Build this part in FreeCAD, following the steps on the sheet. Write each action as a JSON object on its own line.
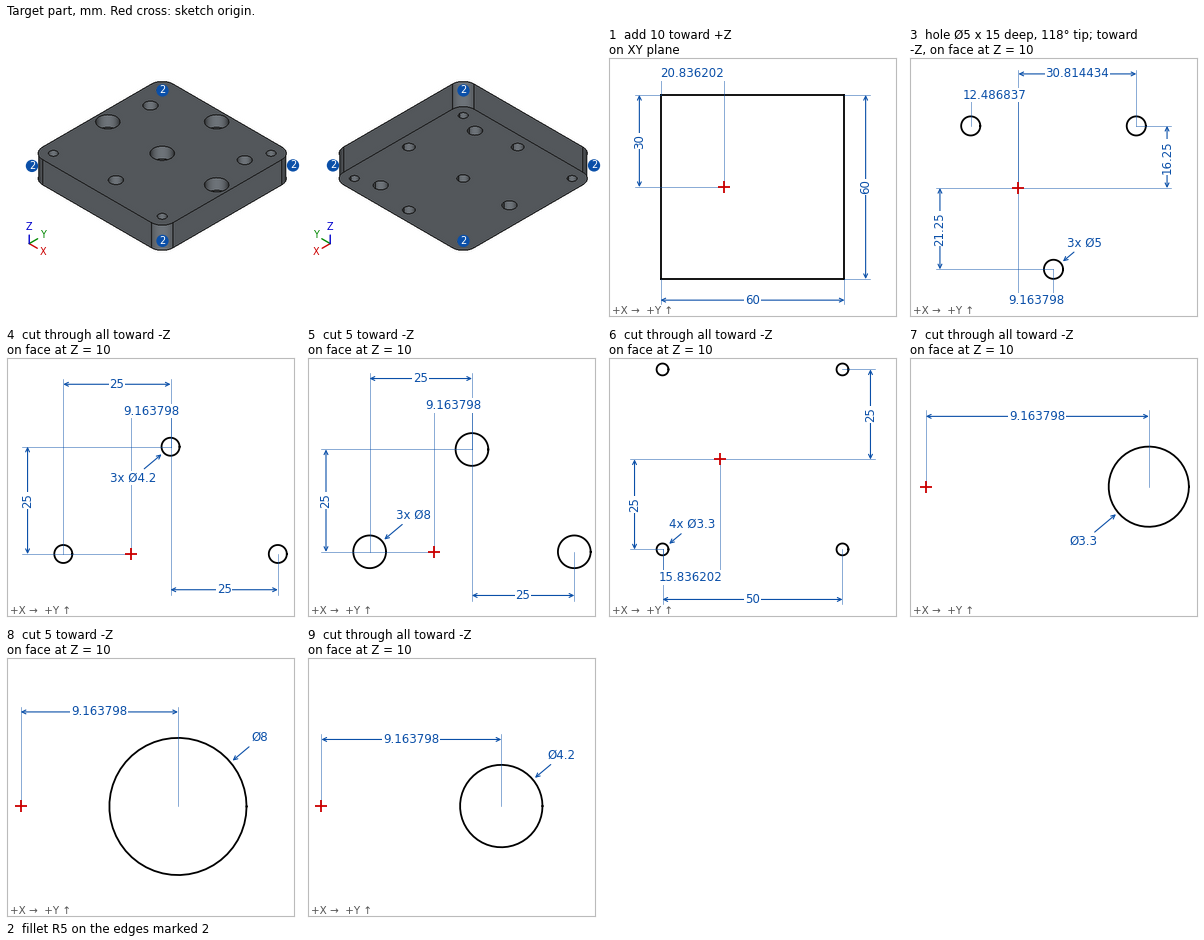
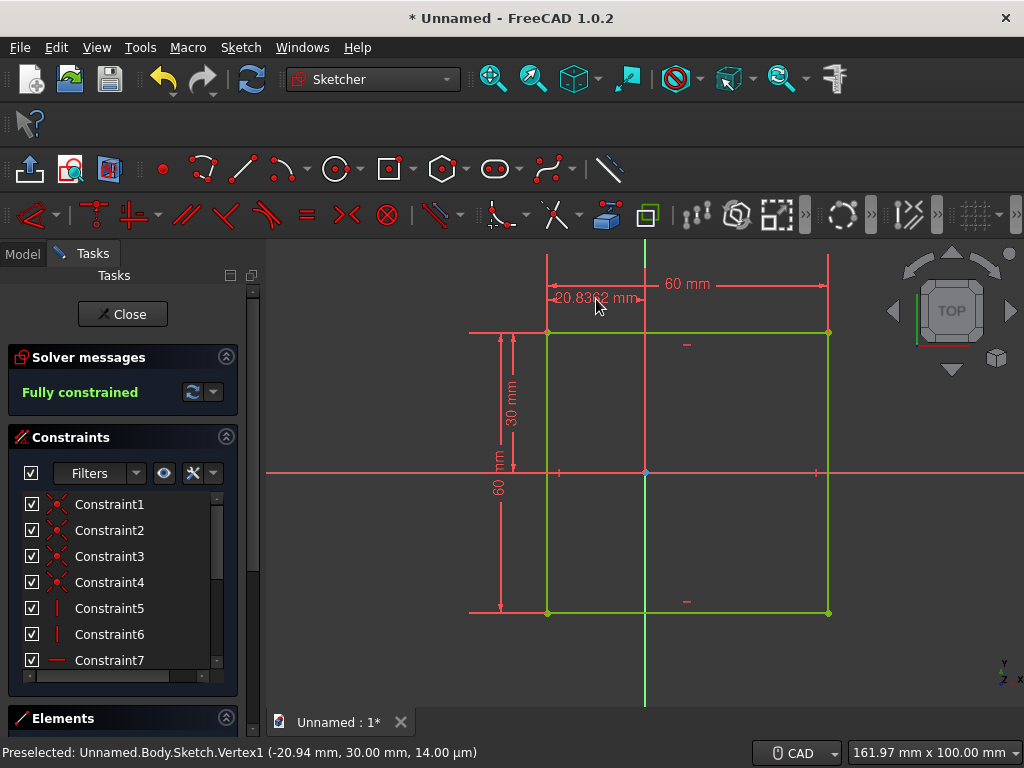
{"action": "left_click", "coordinate": [123, 314]}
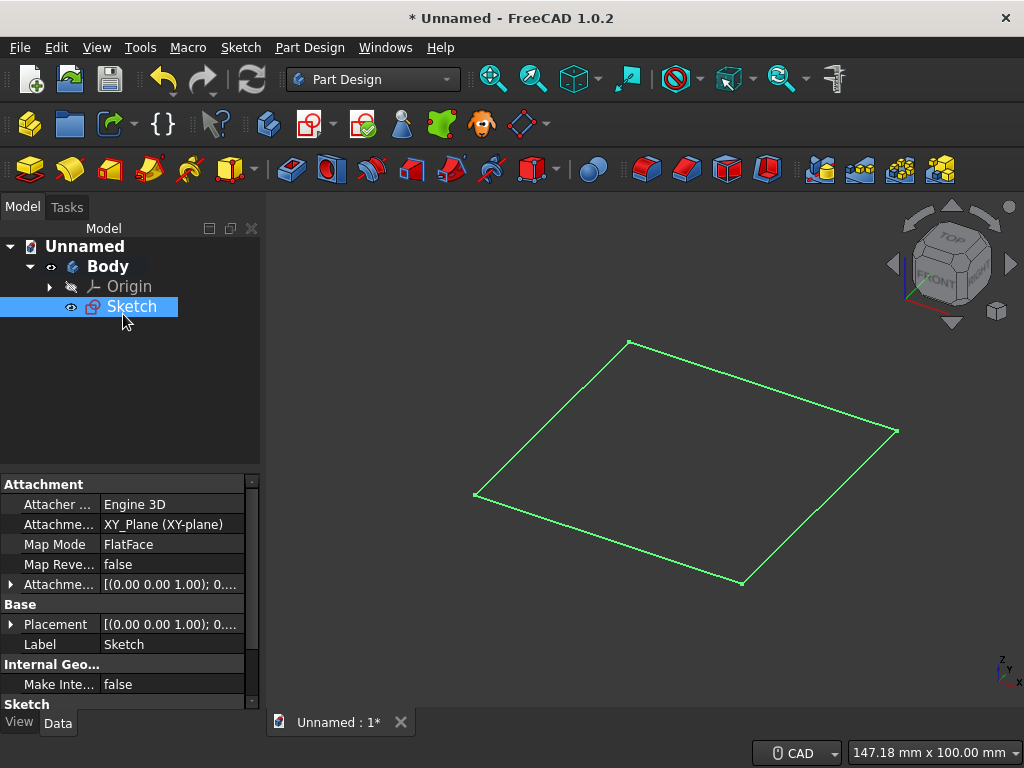
{"action": "left_click", "coordinate": [30, 170]}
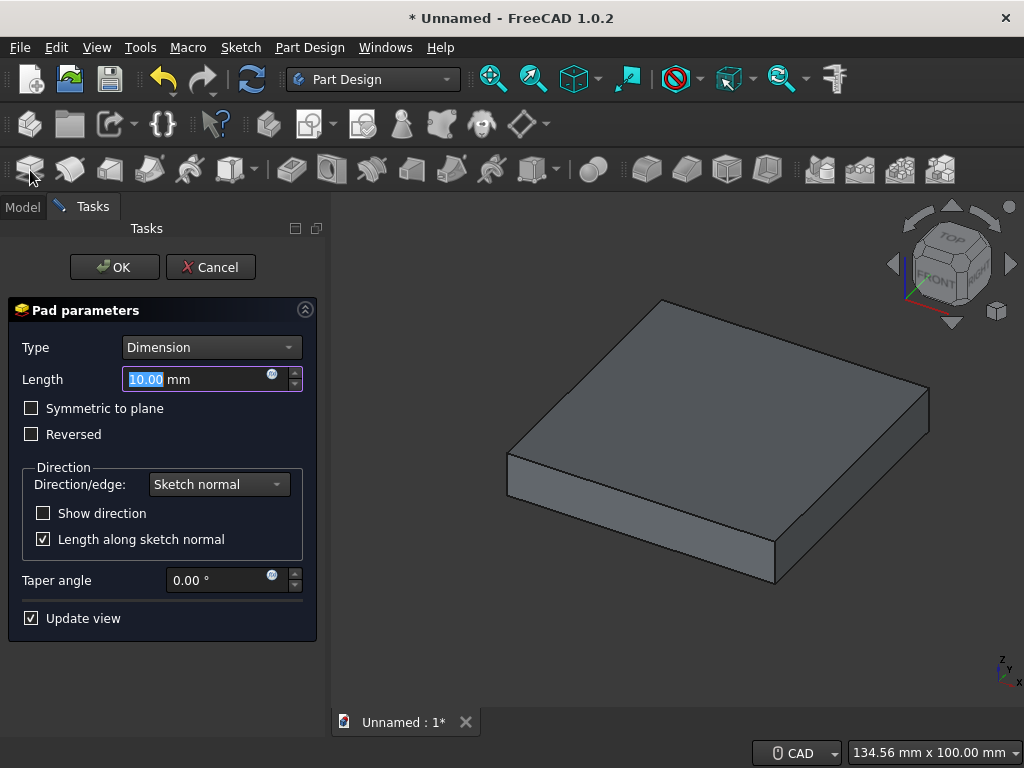
{"action": "type", "text": "10"}
{"action": "key", "text": "Tab"}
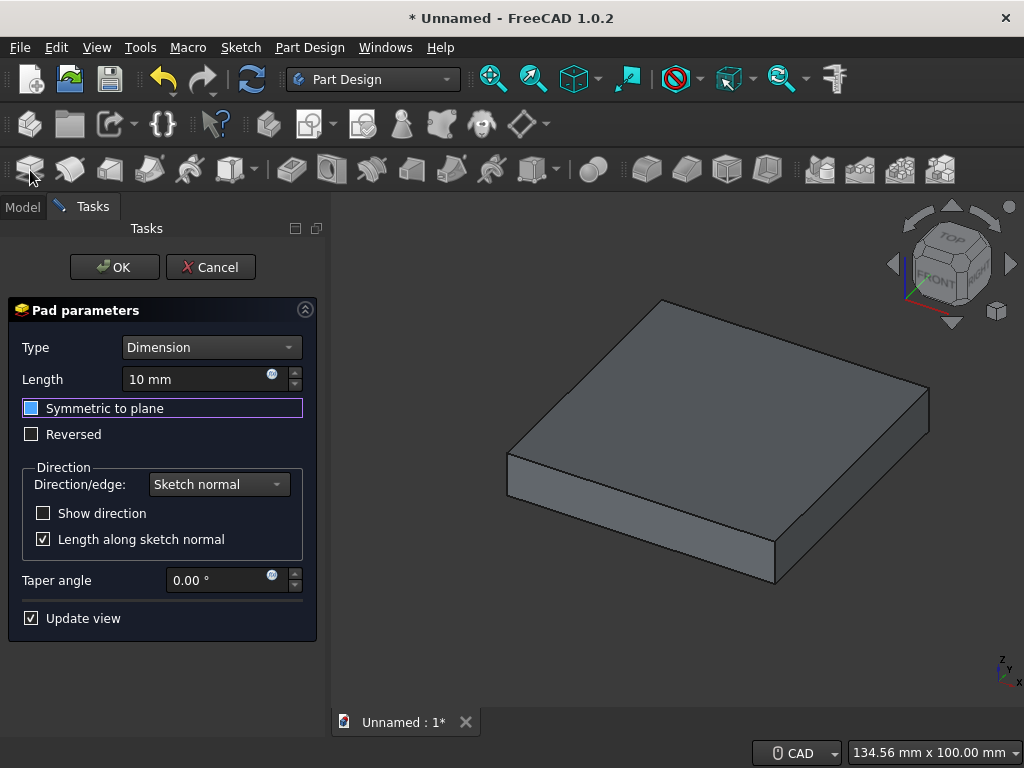
{"action": "left_click", "coordinate": [115, 267]}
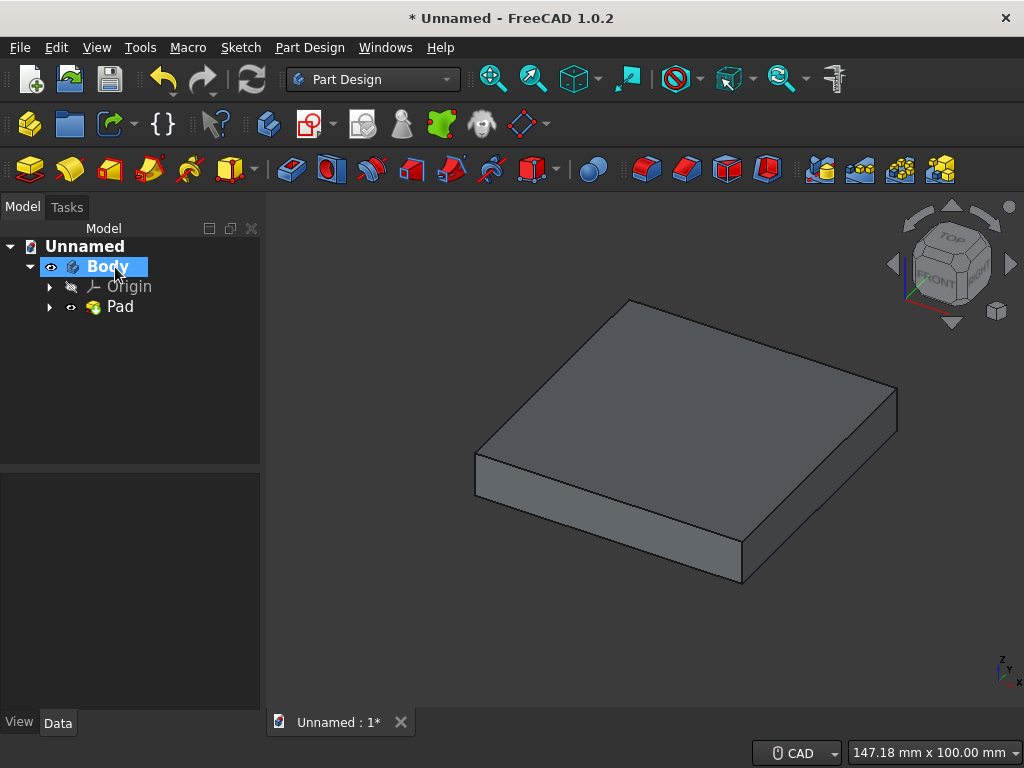
{"action": "left_click", "coordinate": [742, 562]}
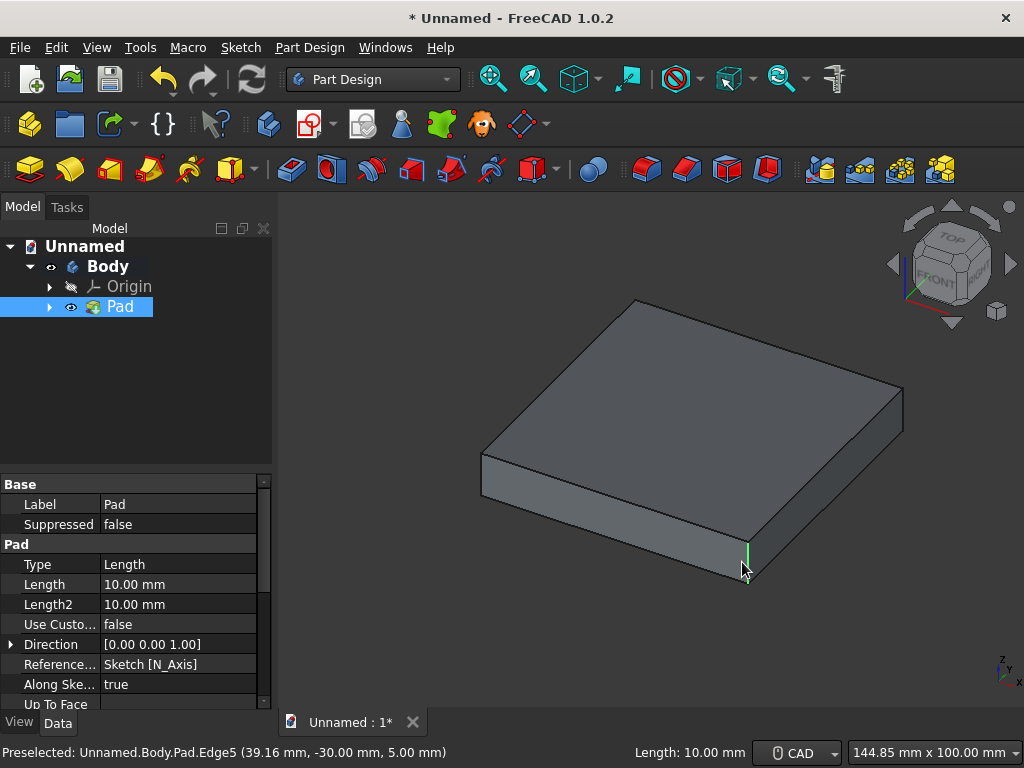
{"action": "key", "text": "0"}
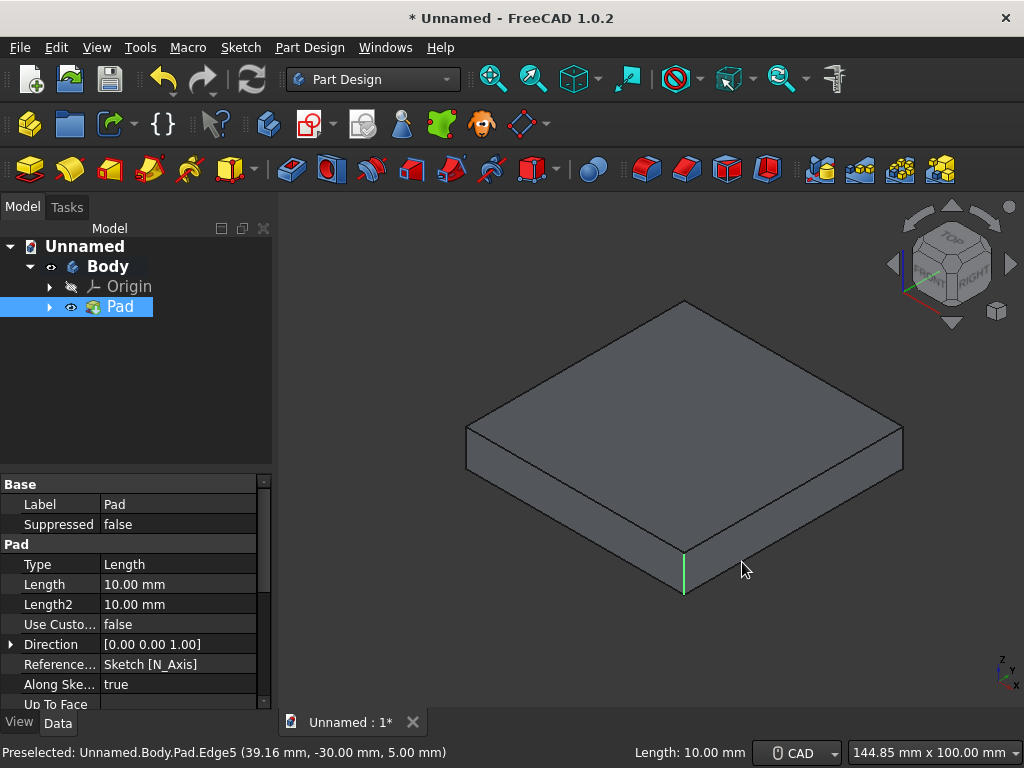
{"action": "key", "text": "2"}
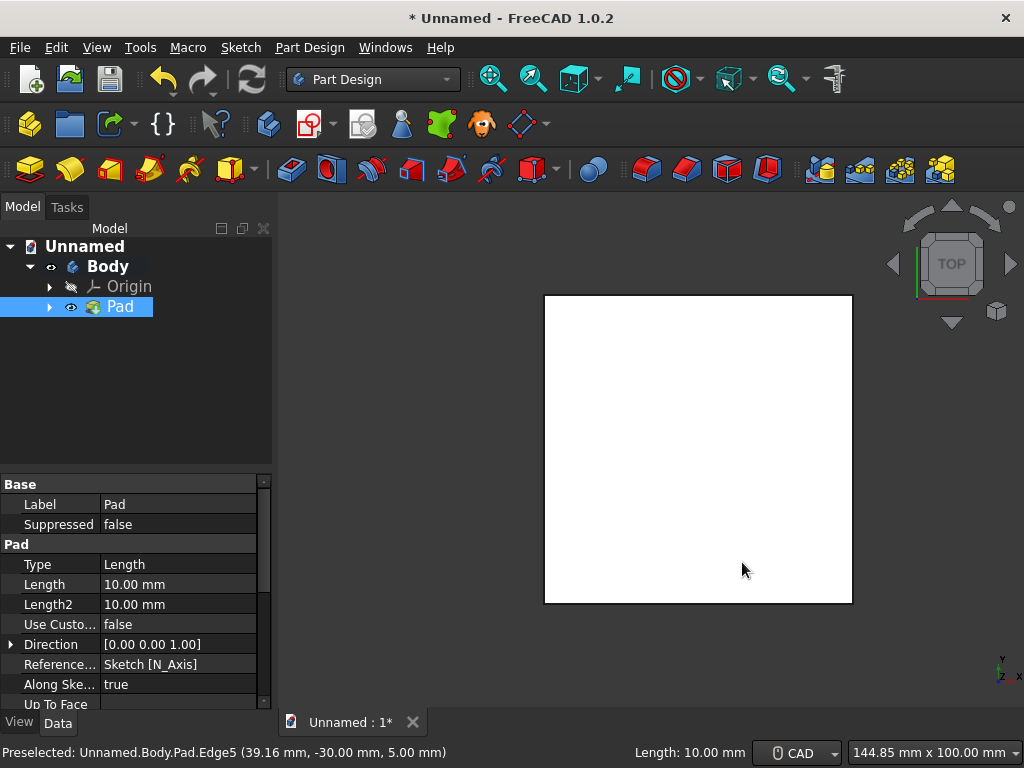
{"action": "key", "text": "1"}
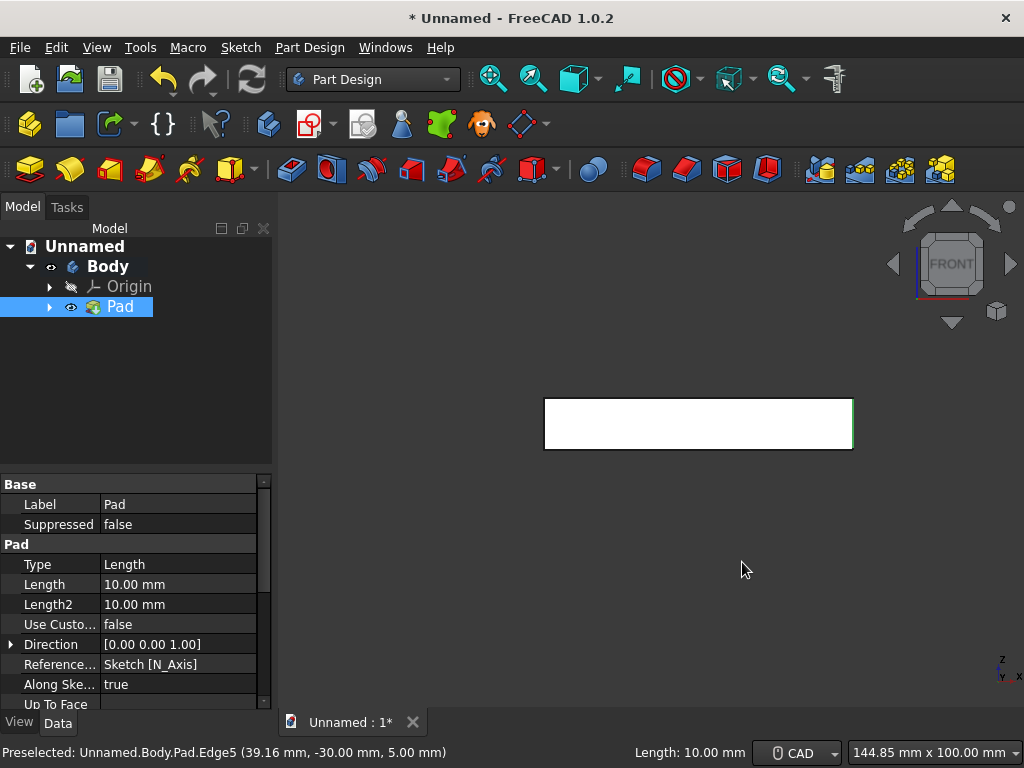
{"action": "left_click", "coordinate": [494, 80]}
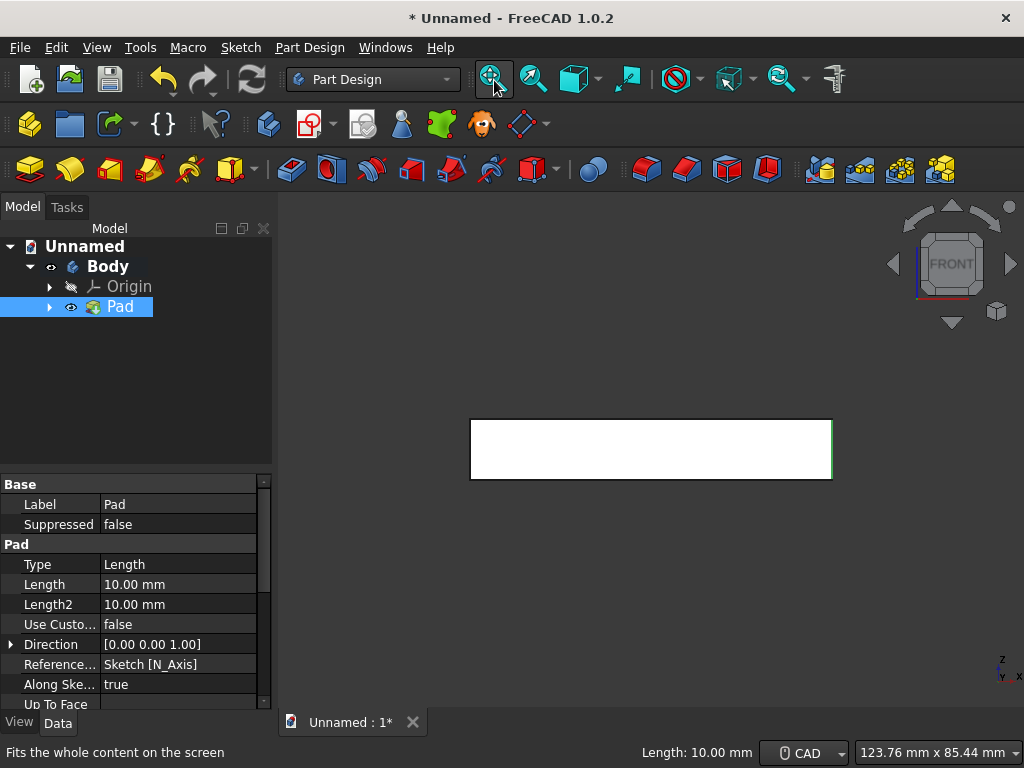
{"action": "left_click", "coordinate": [470, 449], "text": "ctrl"}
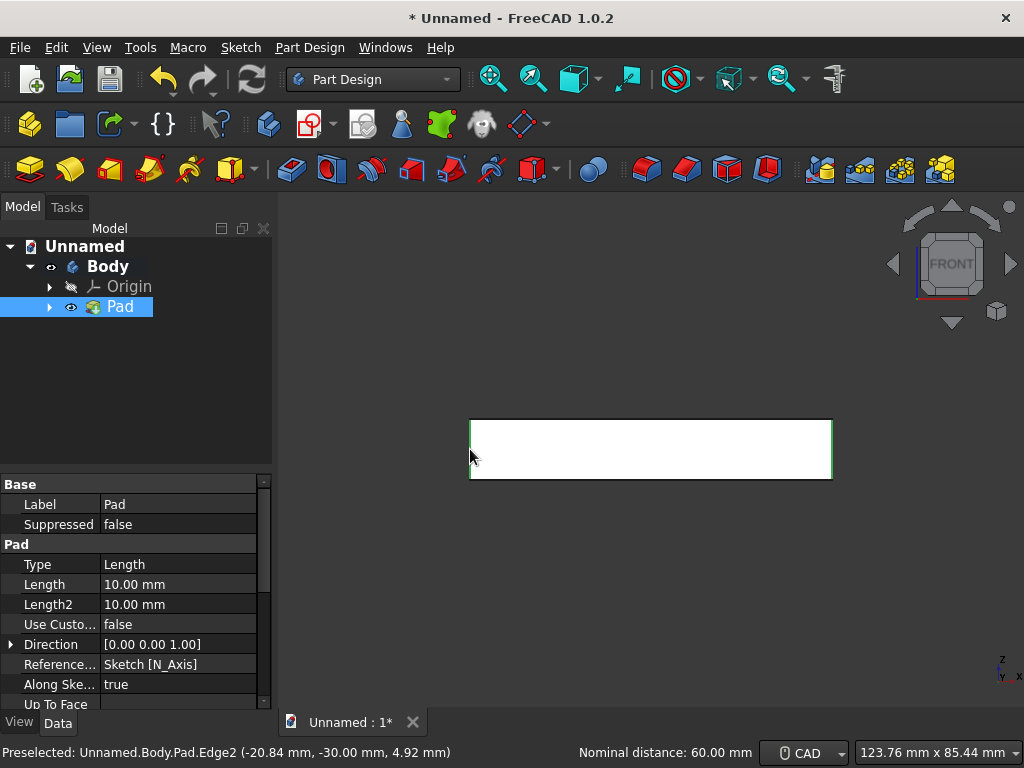
{"action": "key", "text": "3"}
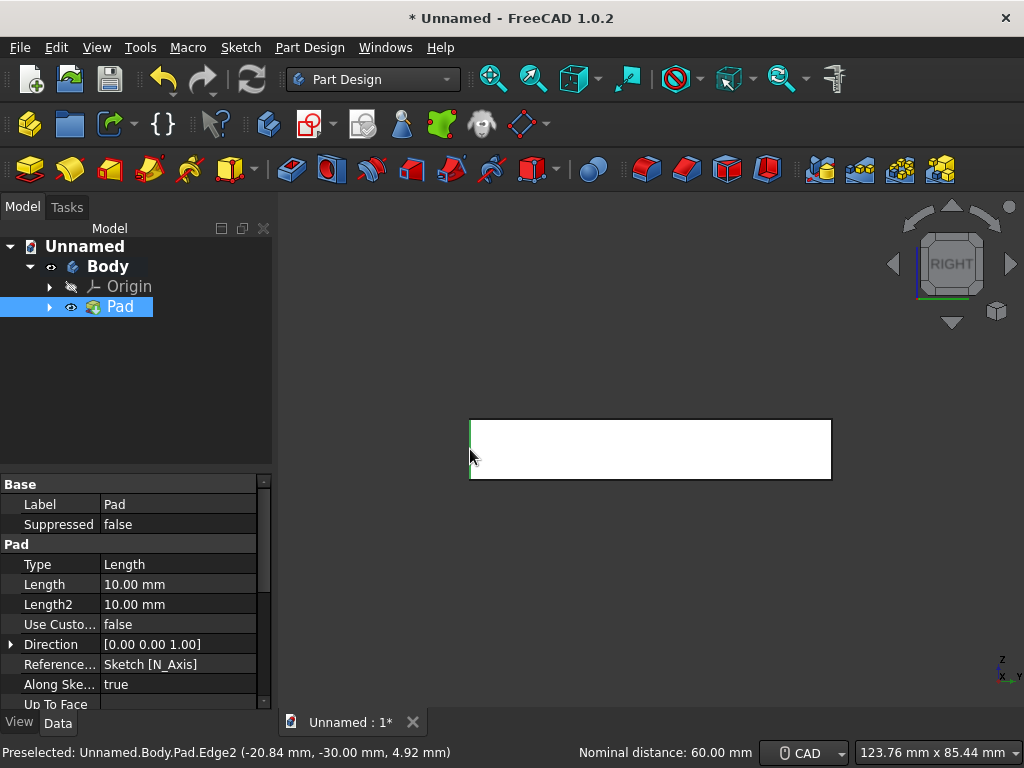
{"action": "left_click", "coordinate": [832, 448], "text": "ctrl"}